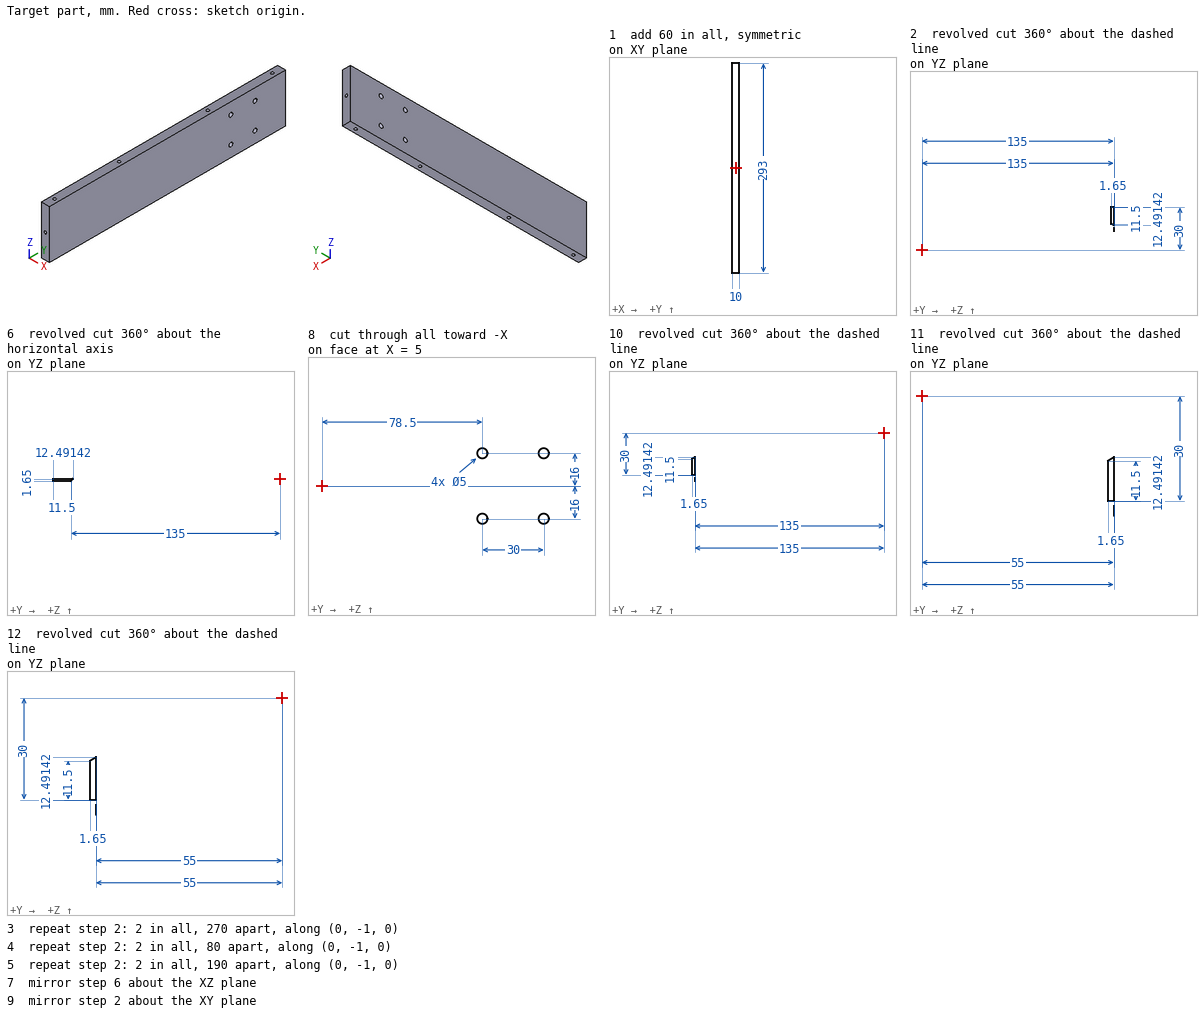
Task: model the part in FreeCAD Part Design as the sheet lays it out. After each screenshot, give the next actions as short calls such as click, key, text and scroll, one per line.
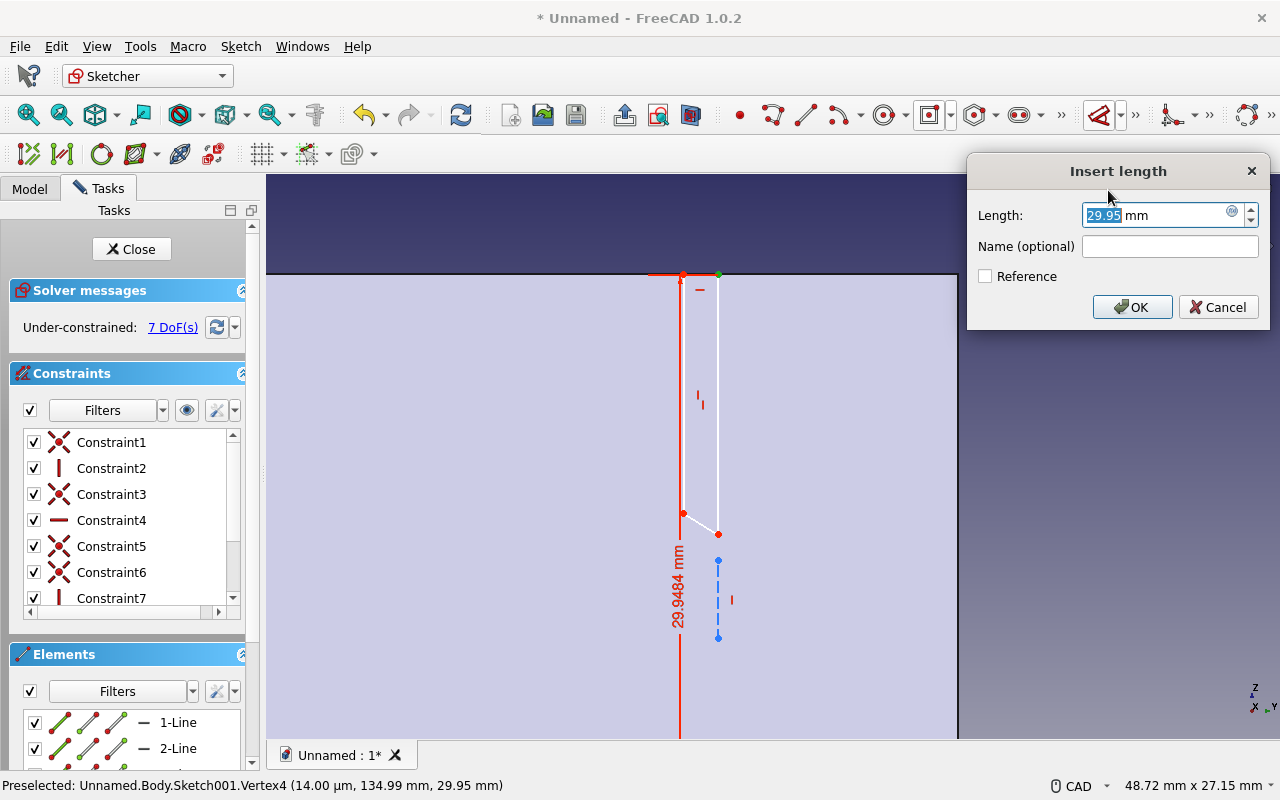
text(30)
key(Return)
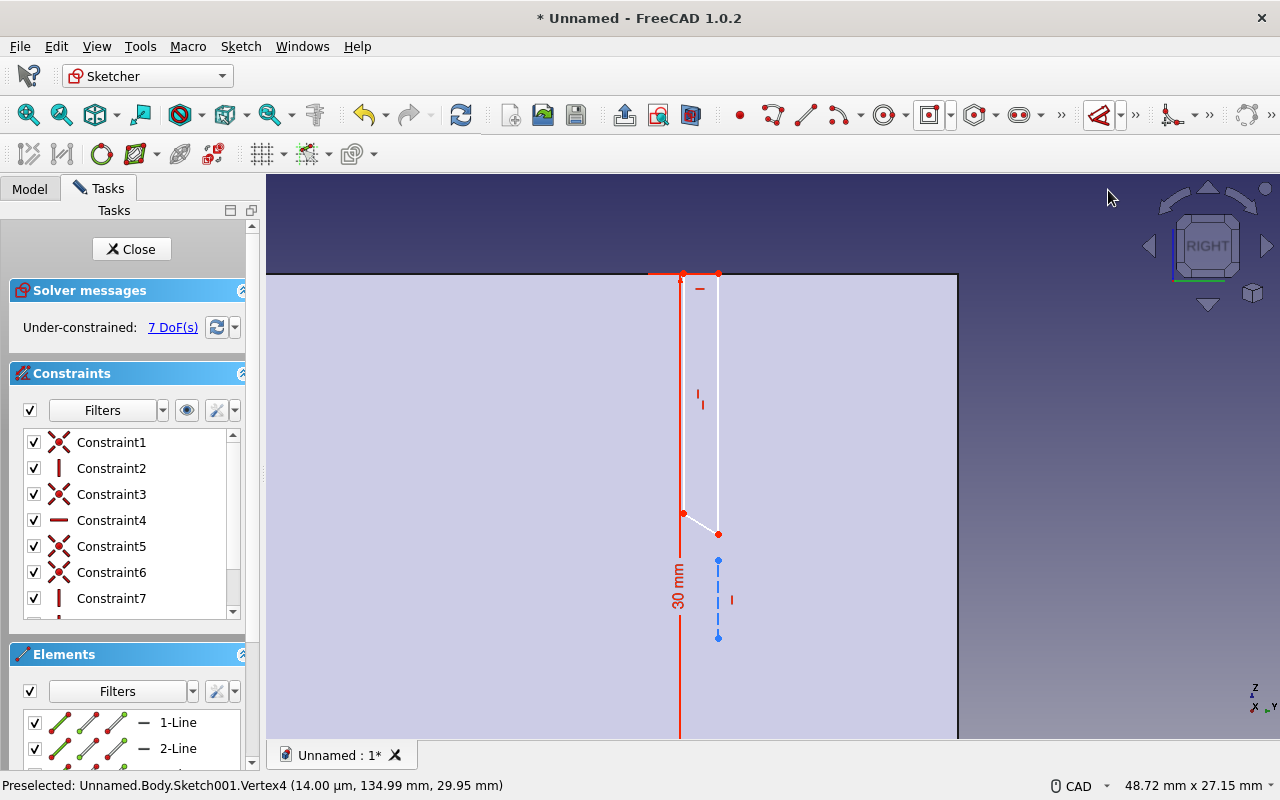
scroll(708, 274, up, 2)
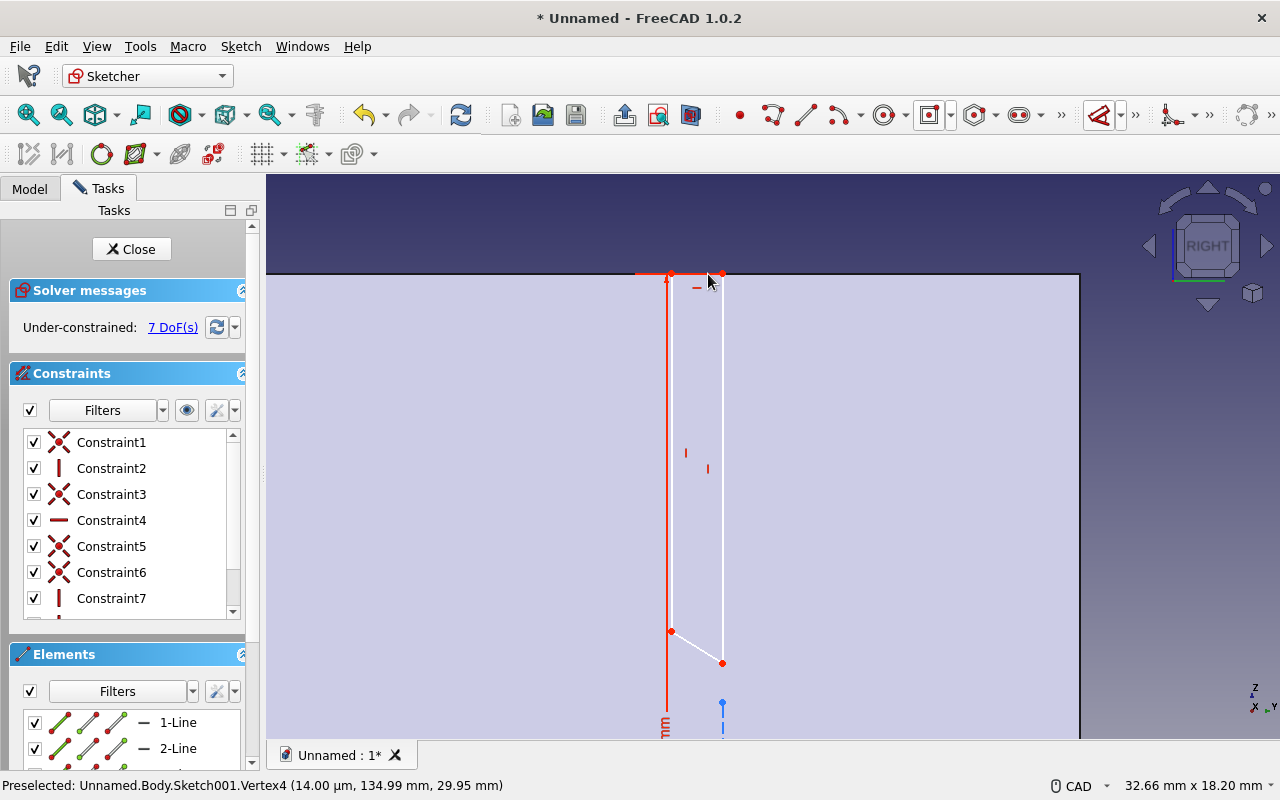
click(707, 274)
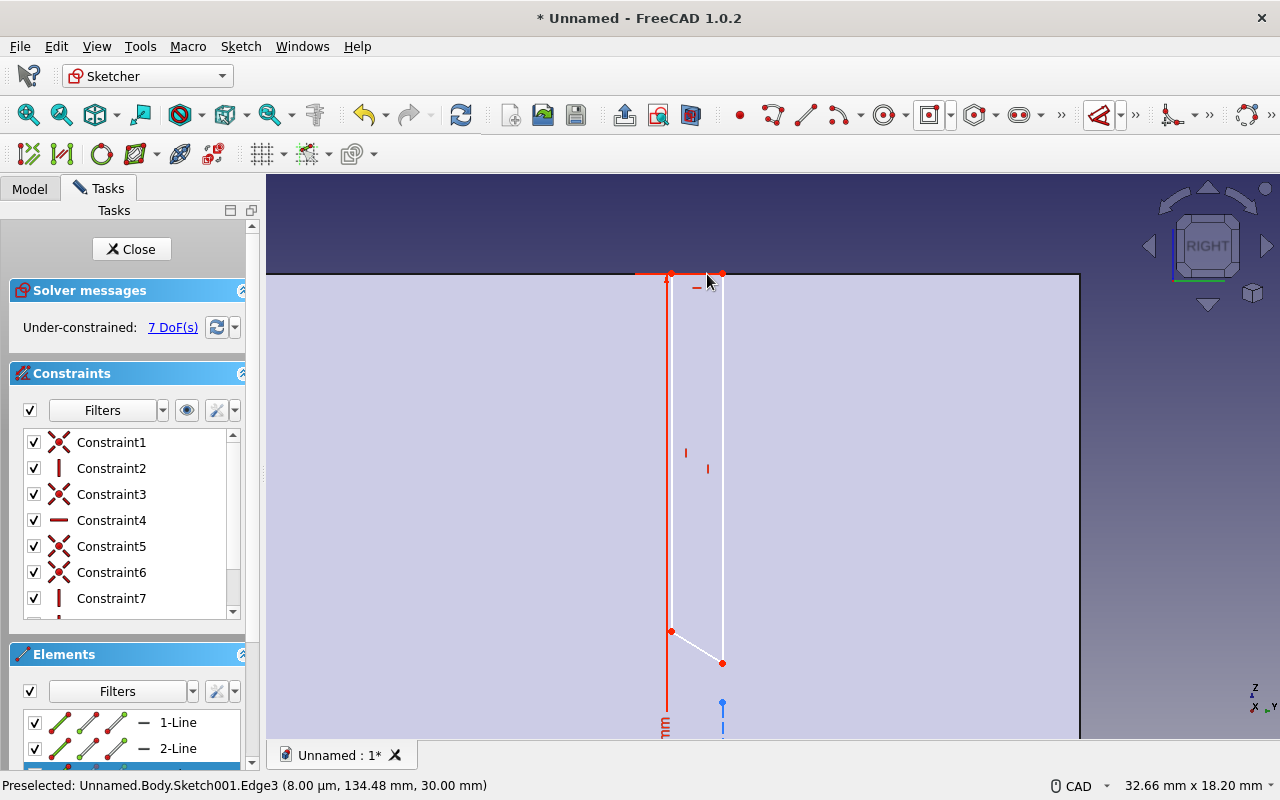
key(l)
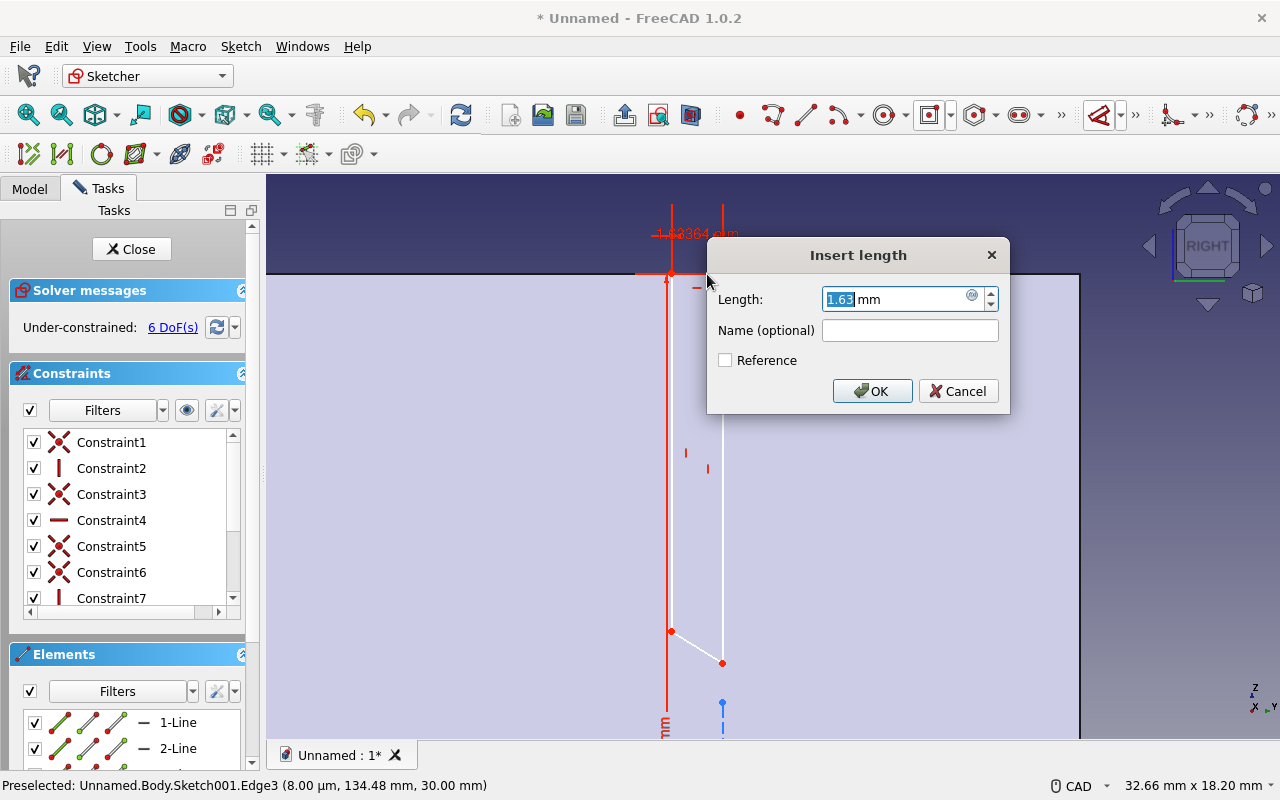
text(1.65)
key(Return)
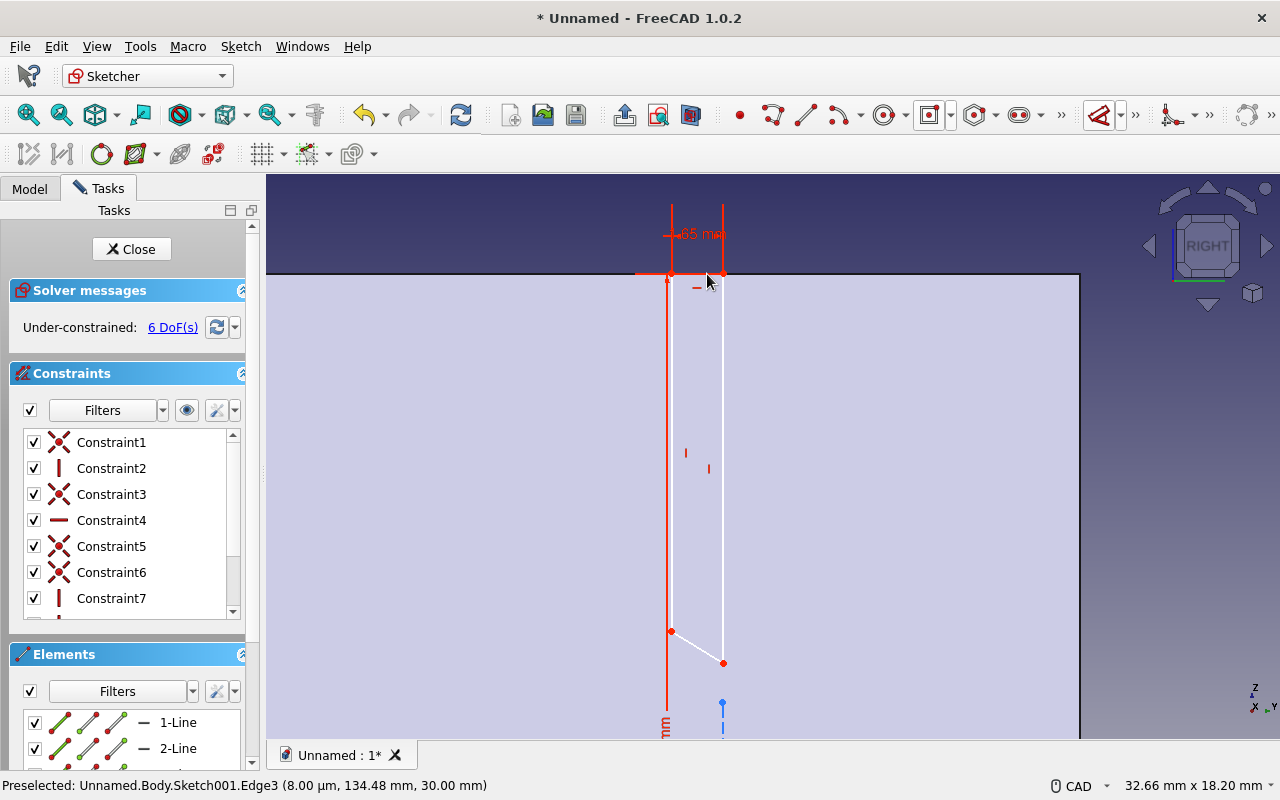
click(672, 381)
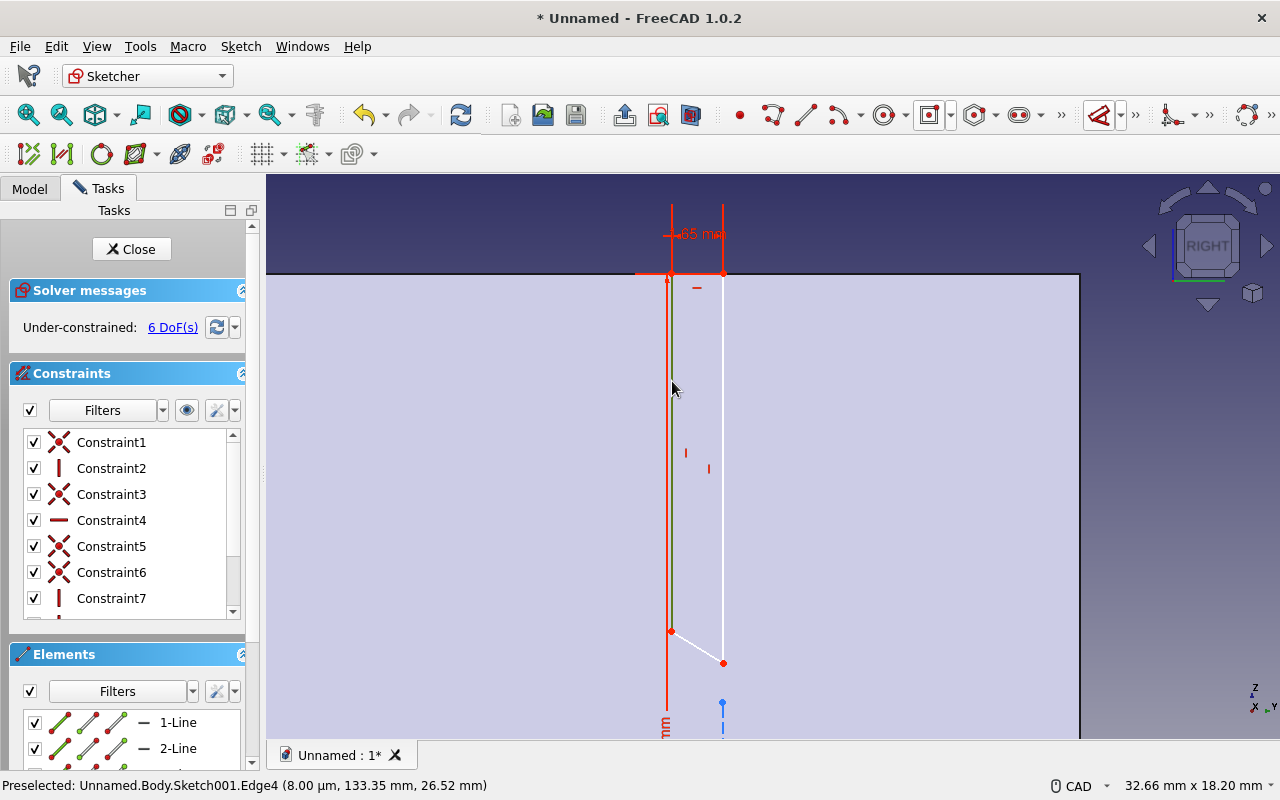
key(i)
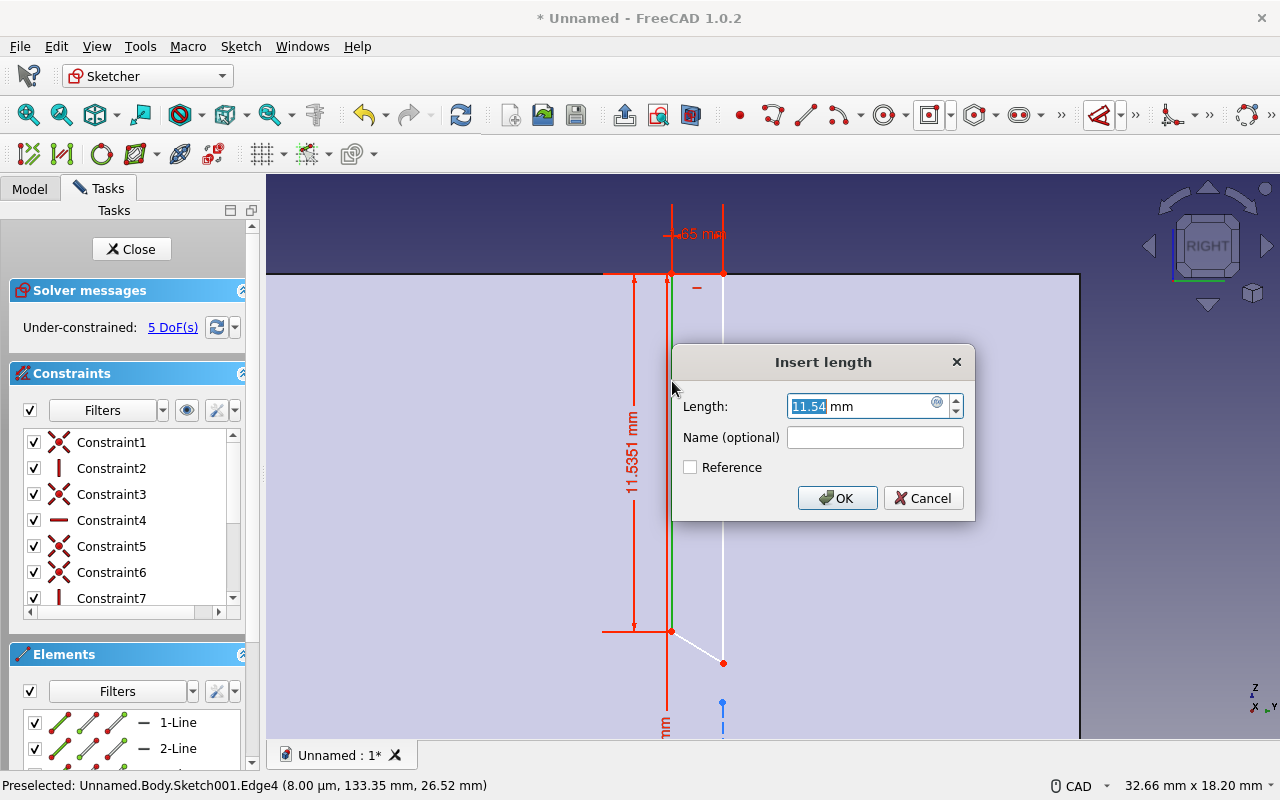
text(11.5)
key(Return)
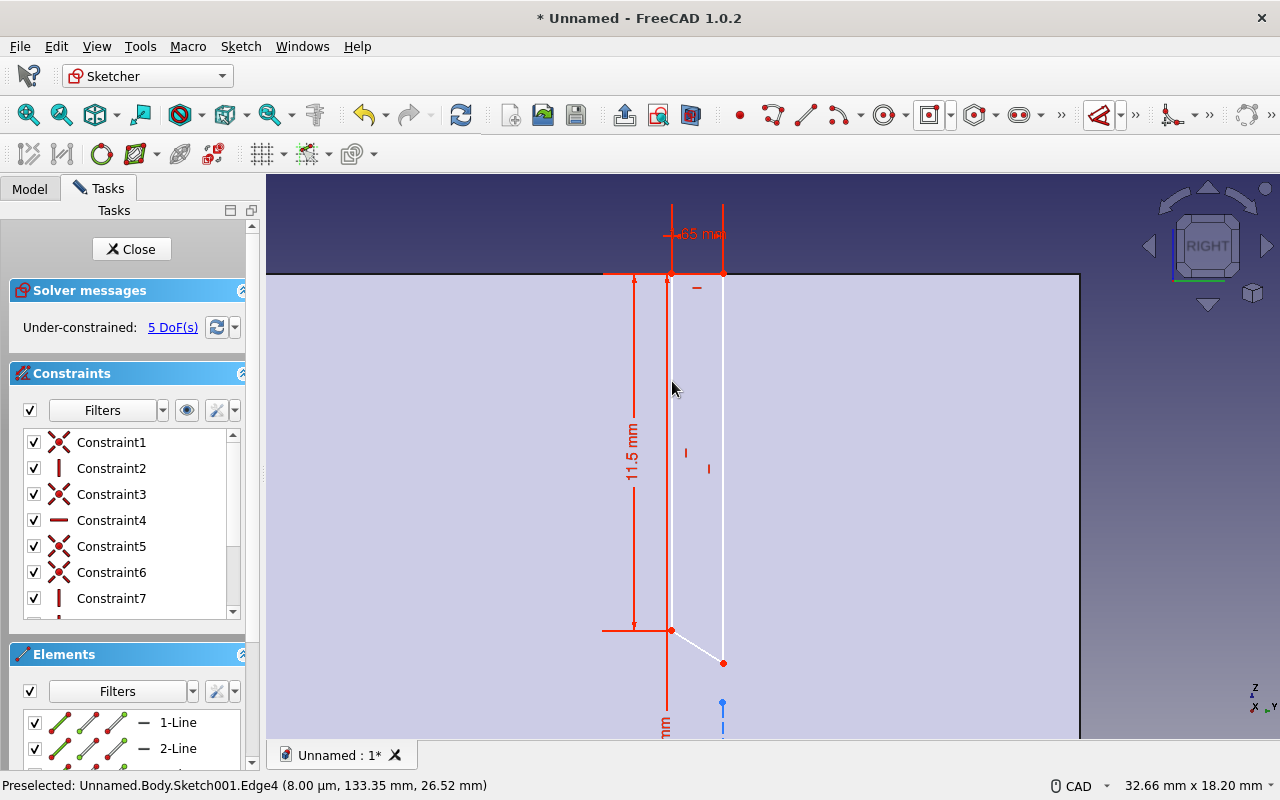
click(723, 663)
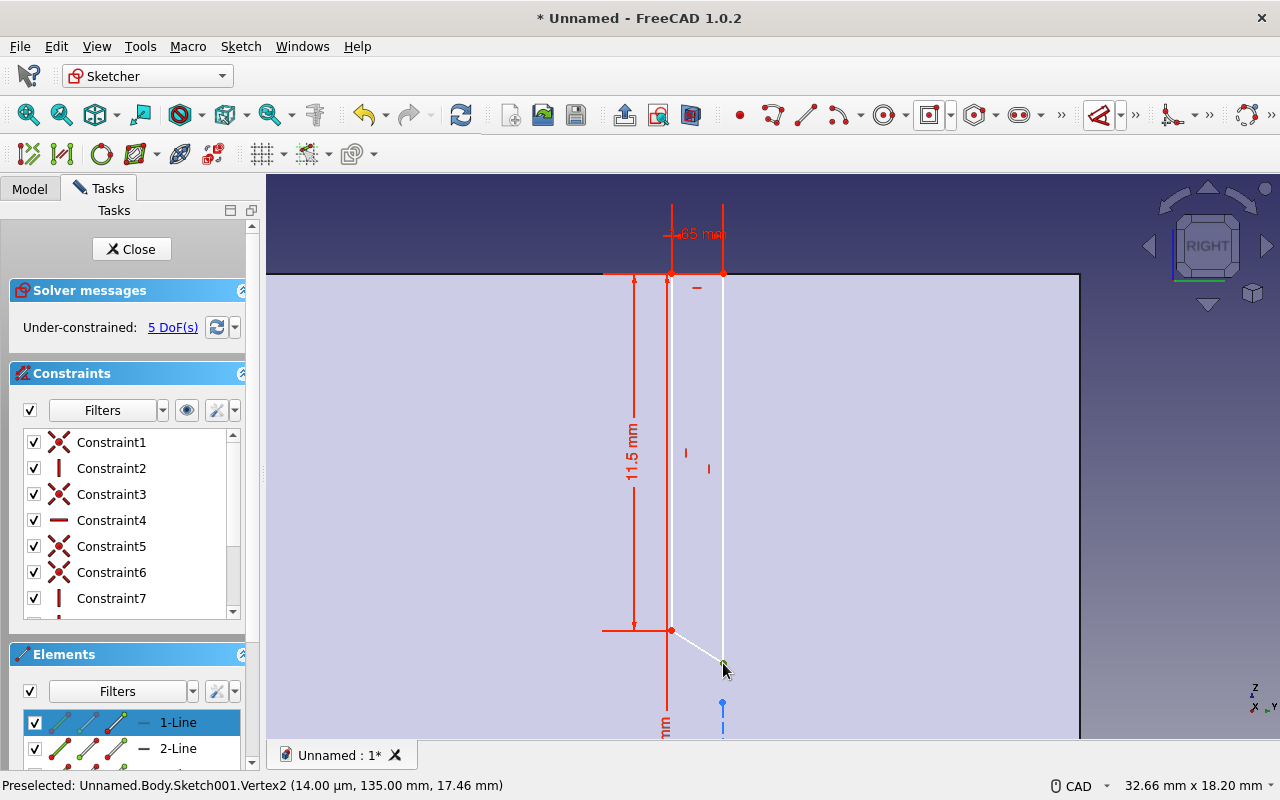
key(l)